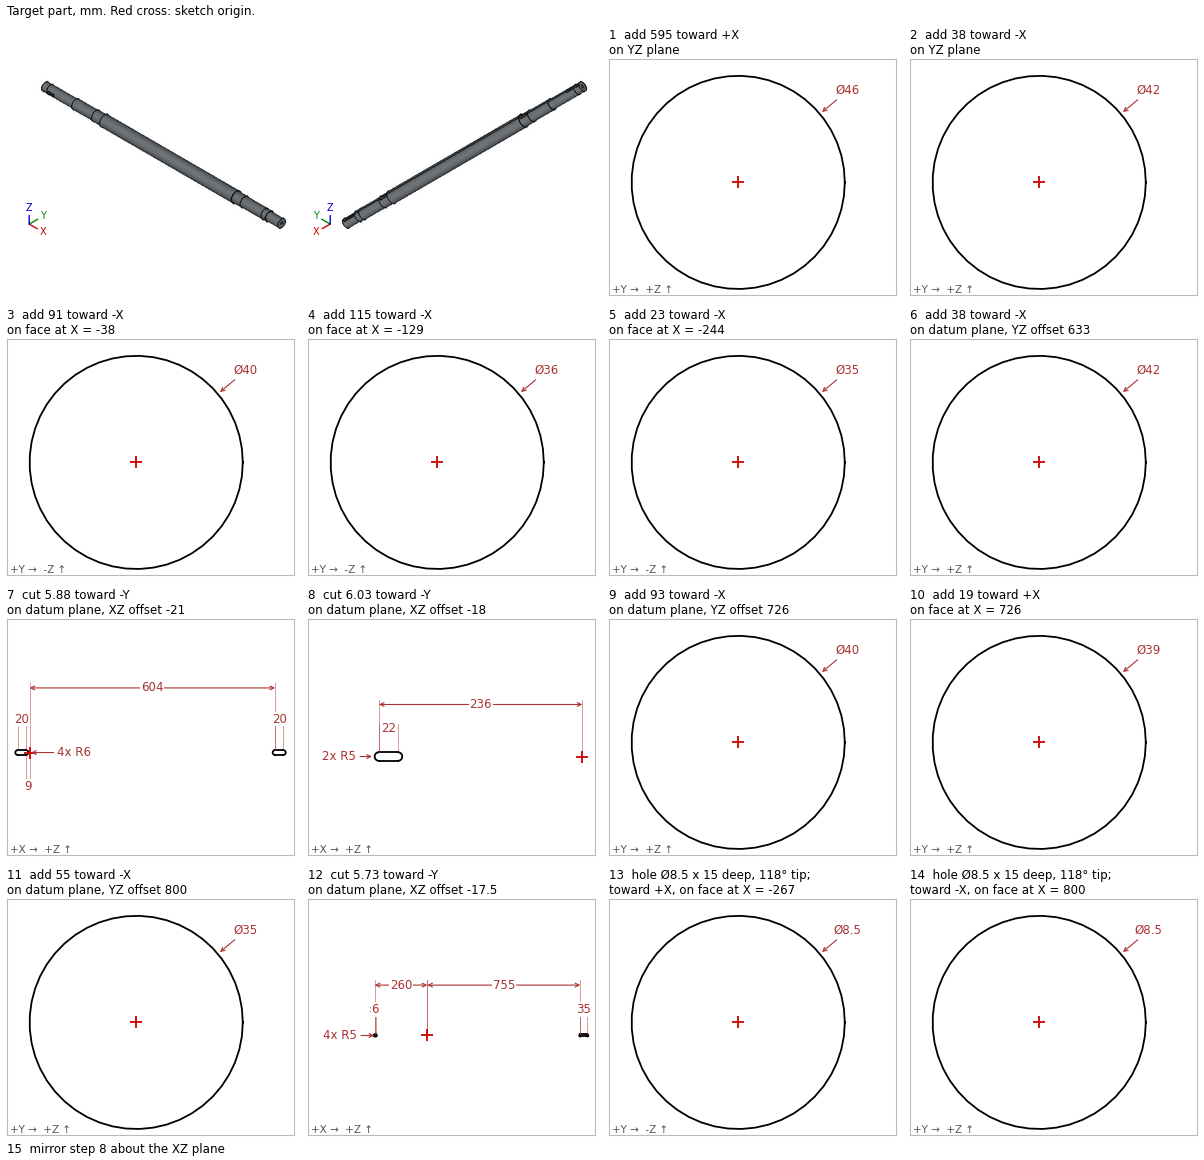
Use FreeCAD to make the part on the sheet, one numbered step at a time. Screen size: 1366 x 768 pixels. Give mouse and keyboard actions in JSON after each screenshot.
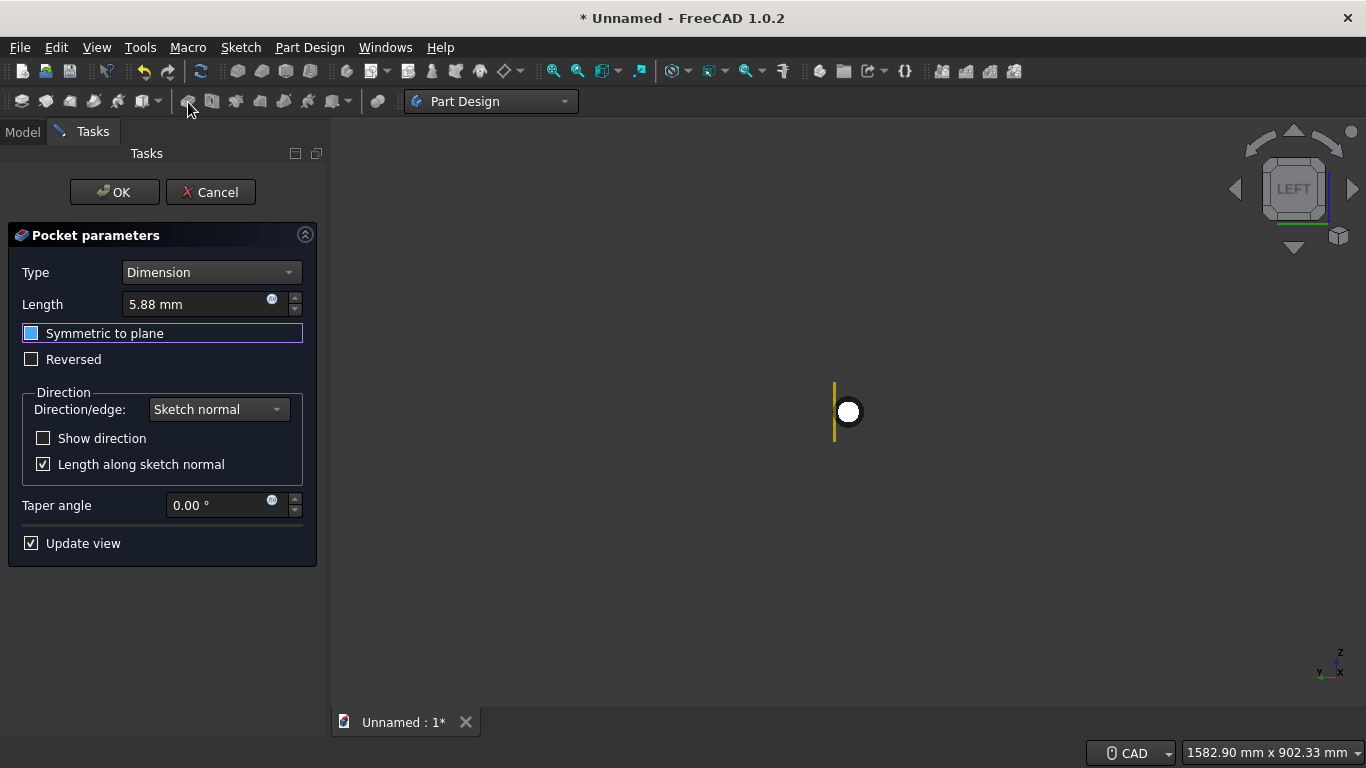
{"action": "left_click", "coordinate": [30, 359]}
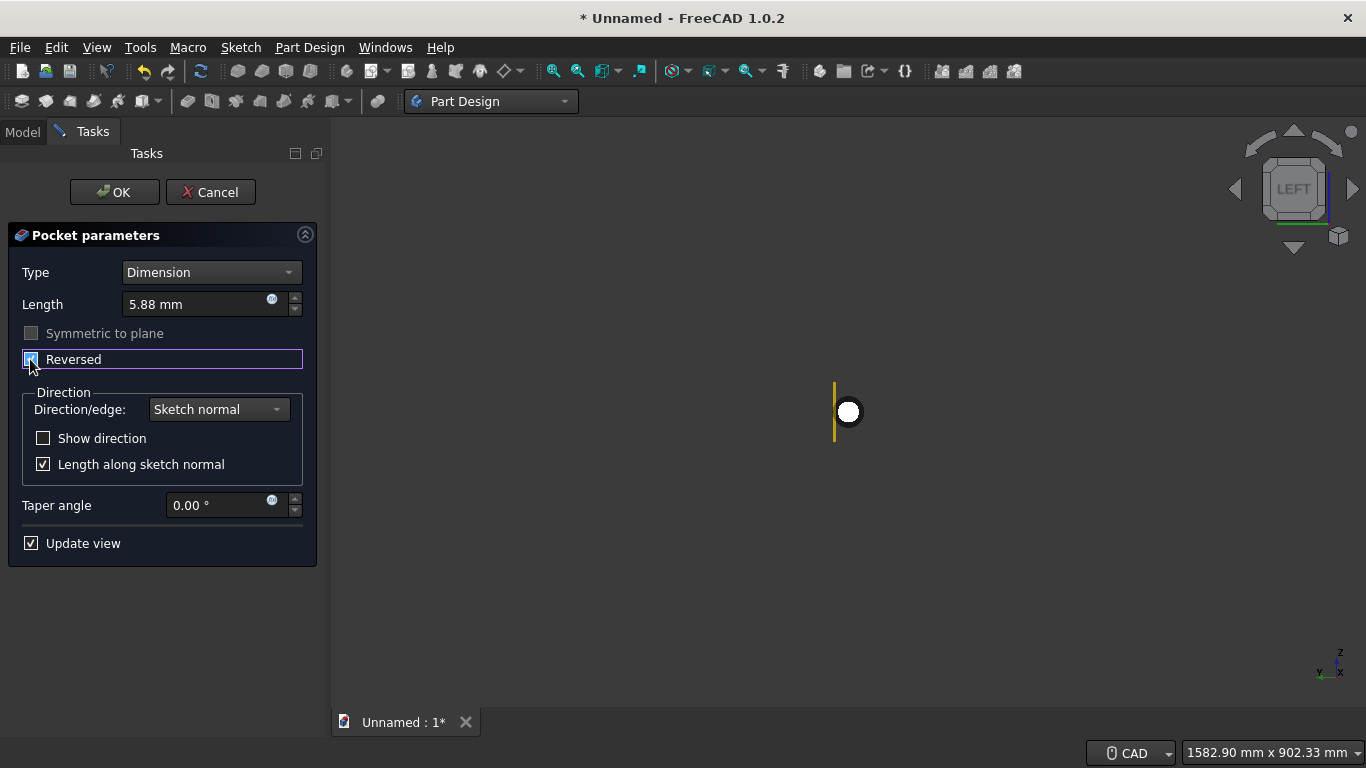
{"action": "left_click", "coordinate": [115, 192]}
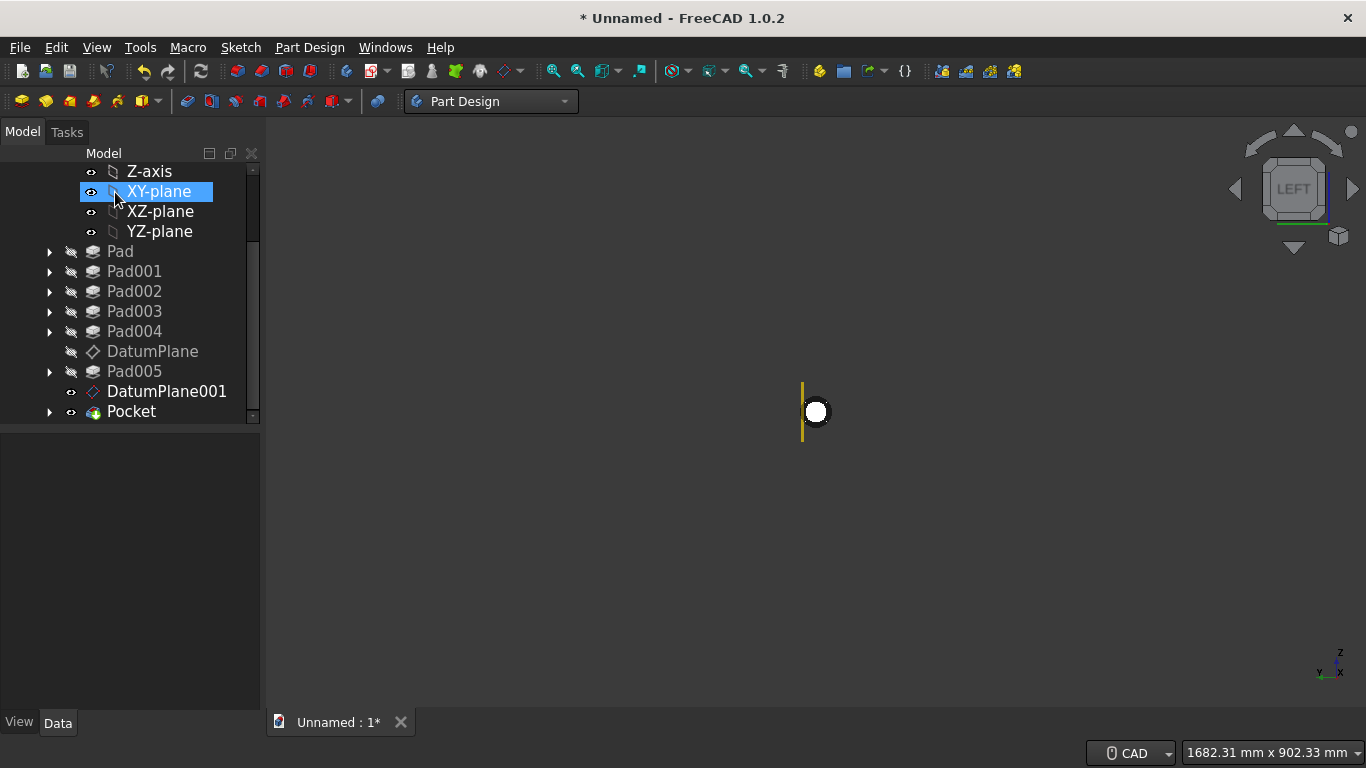
{"action": "left_click", "coordinate": [116, 392]}
{"action": "key", "text": "space"}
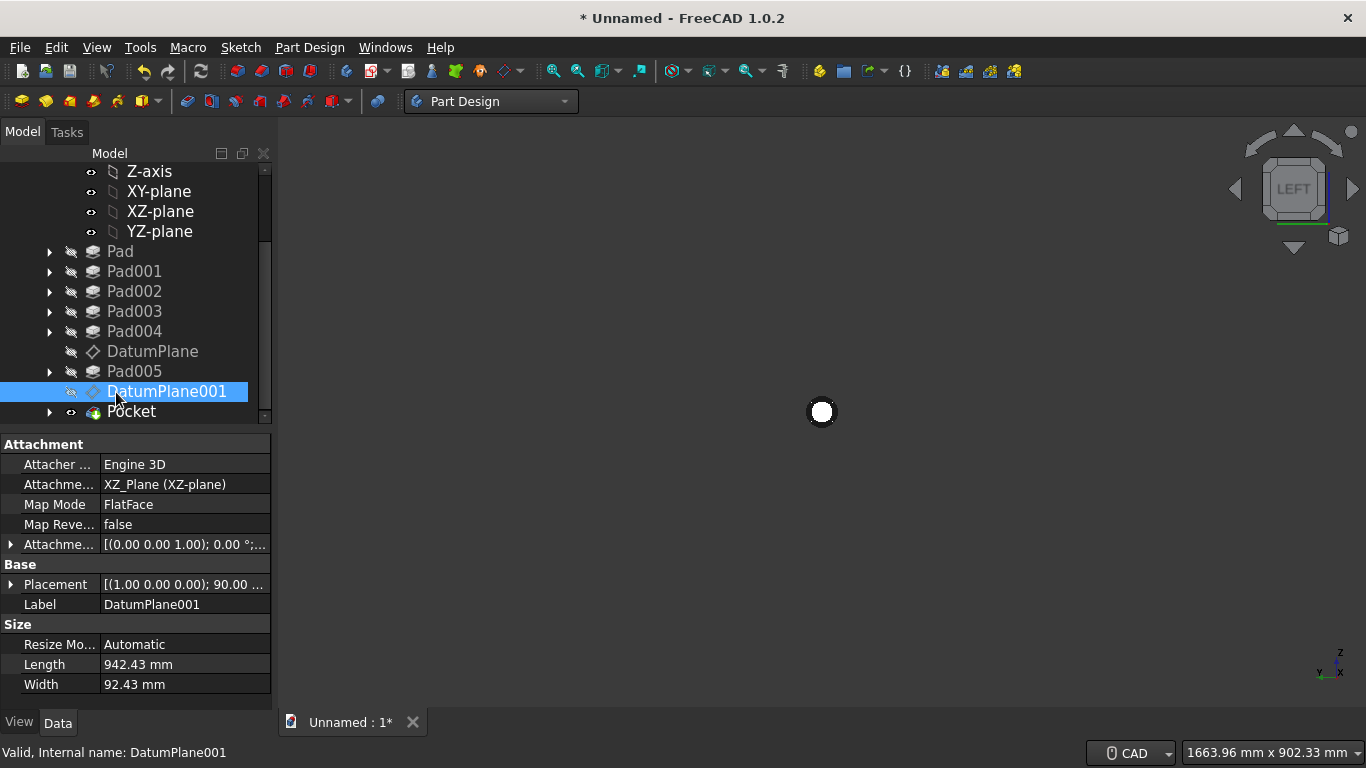
{"action": "left_click", "coordinate": [554, 72]}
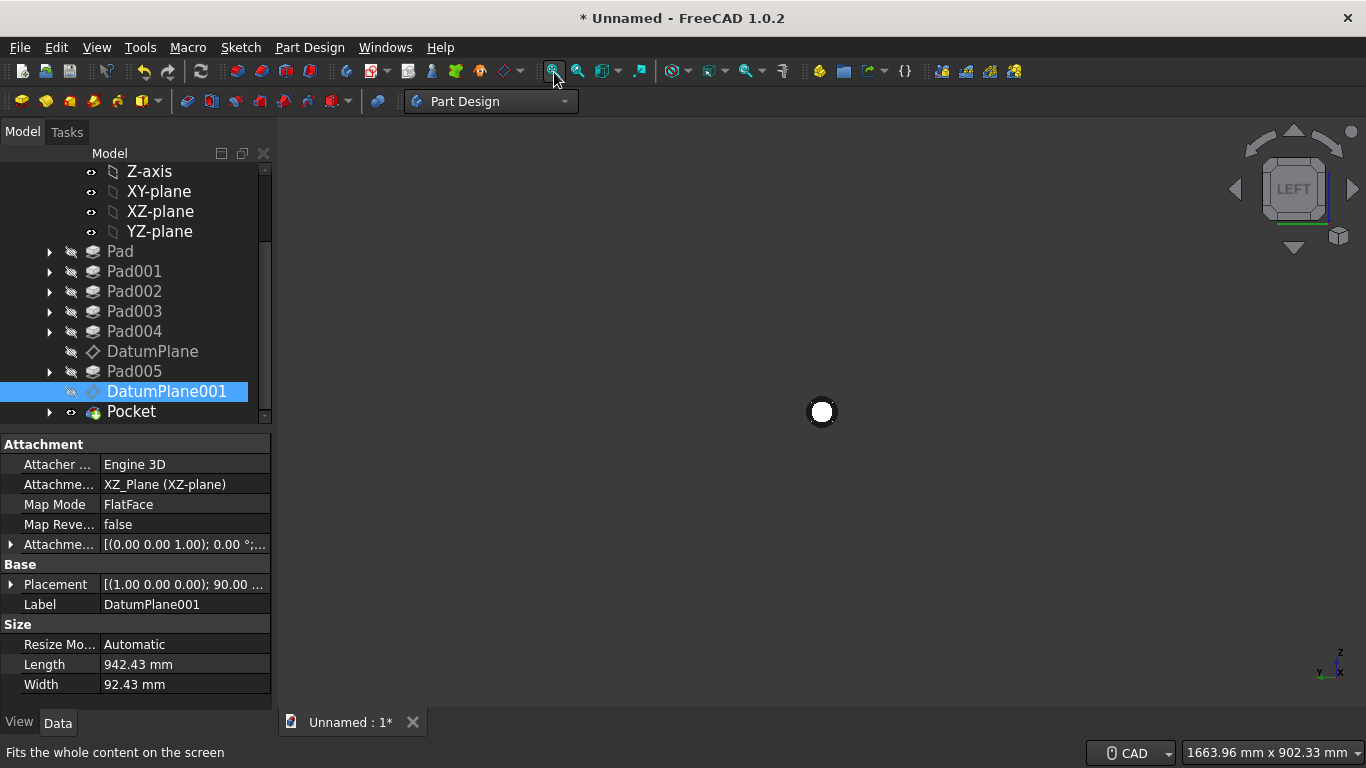
{"action": "scroll", "coordinate": [160, 287], "scroll_direction": "down", "scroll_amount": 3}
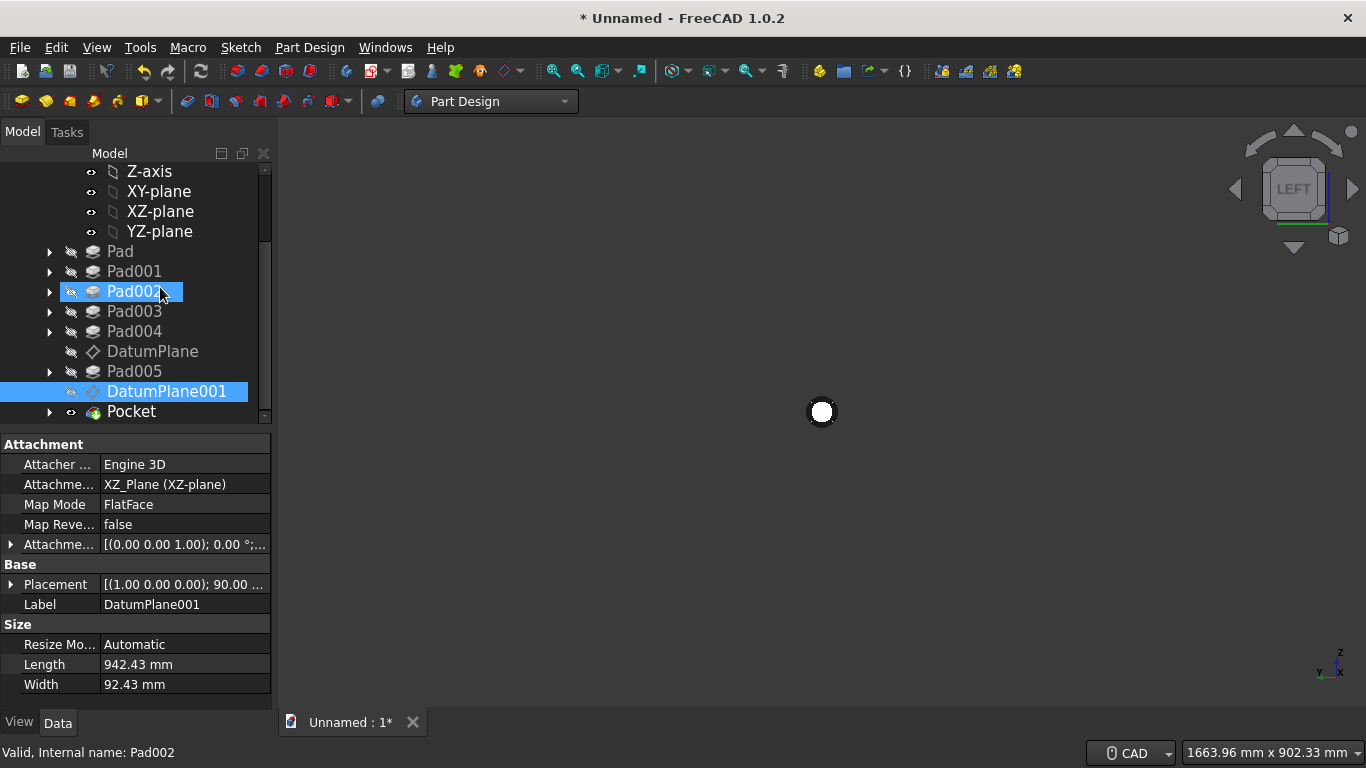
{"action": "scroll", "coordinate": [160, 287], "scroll_direction": "up", "scroll_amount": 15}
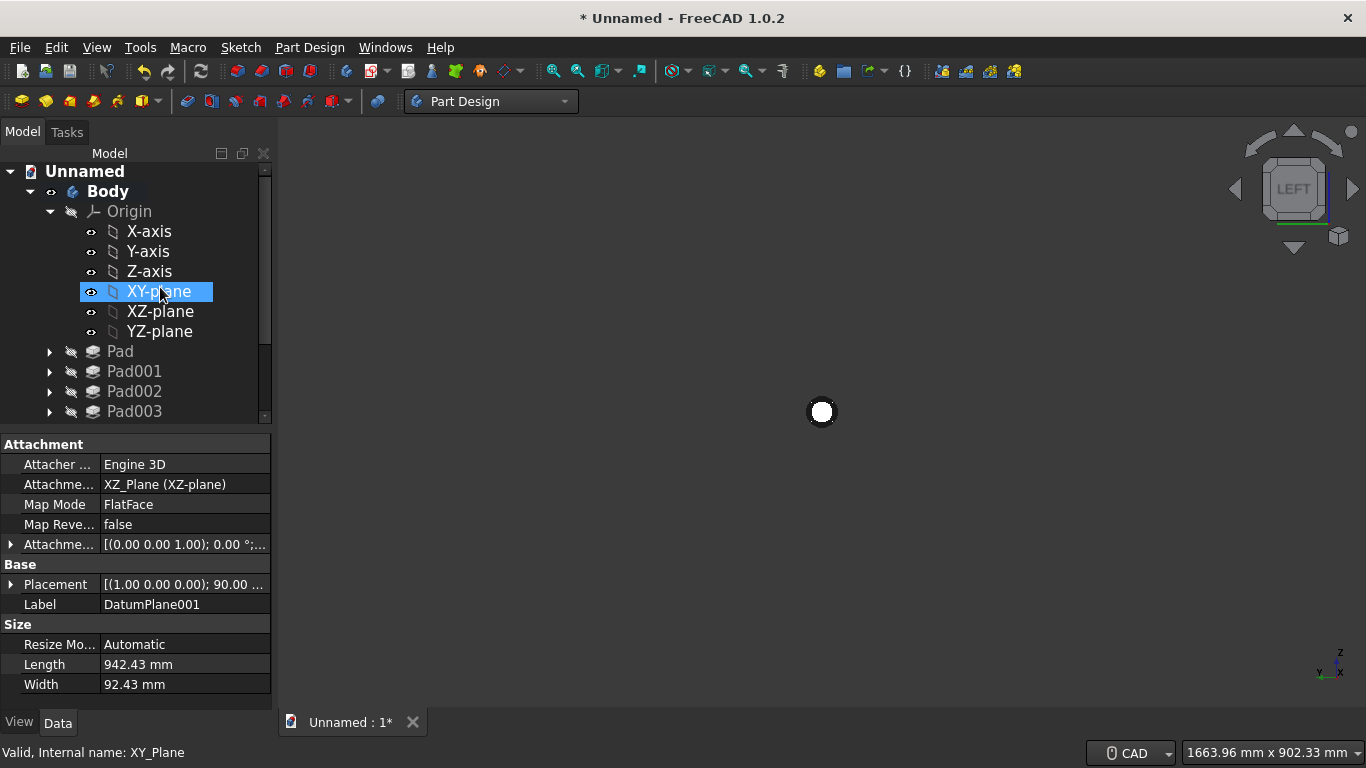
{"action": "left_click", "coordinate": [136, 312]}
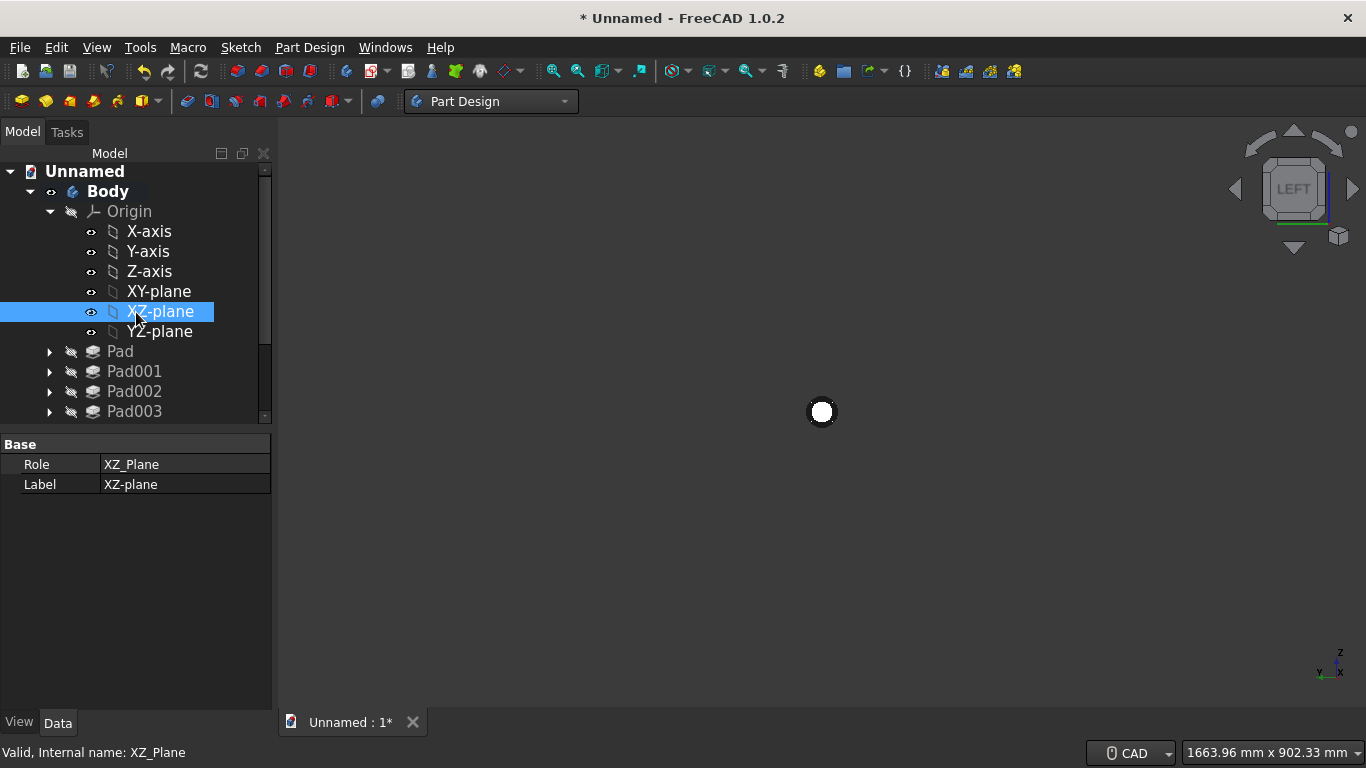
{"action": "left_click", "coordinate": [504, 72]}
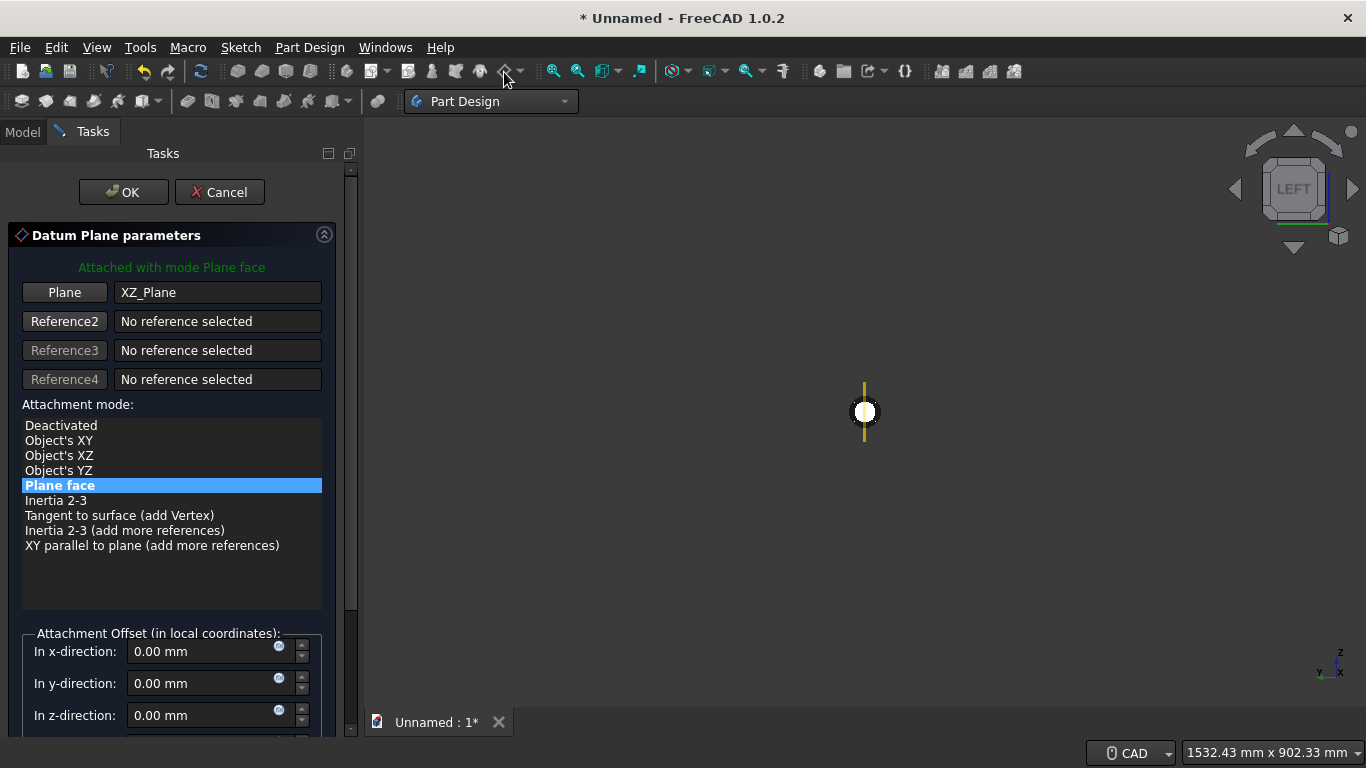
{"action": "triple_click", "coordinate": [210, 715]}